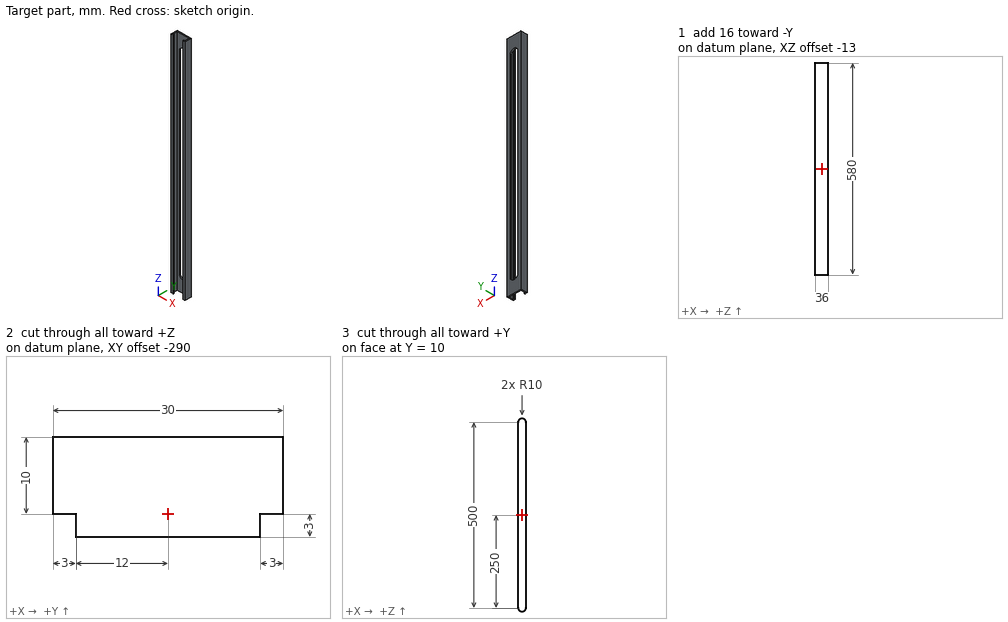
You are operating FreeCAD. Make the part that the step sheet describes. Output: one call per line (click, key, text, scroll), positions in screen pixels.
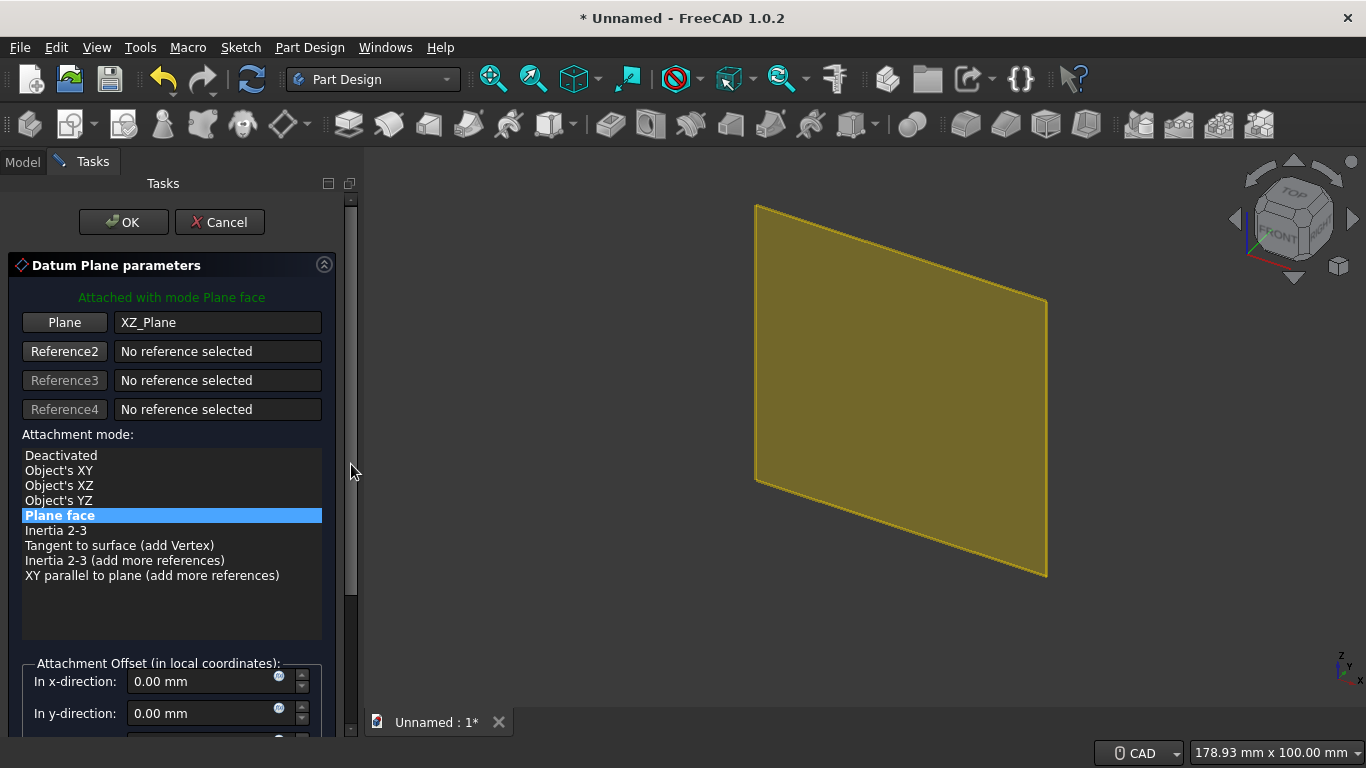
click(124, 222)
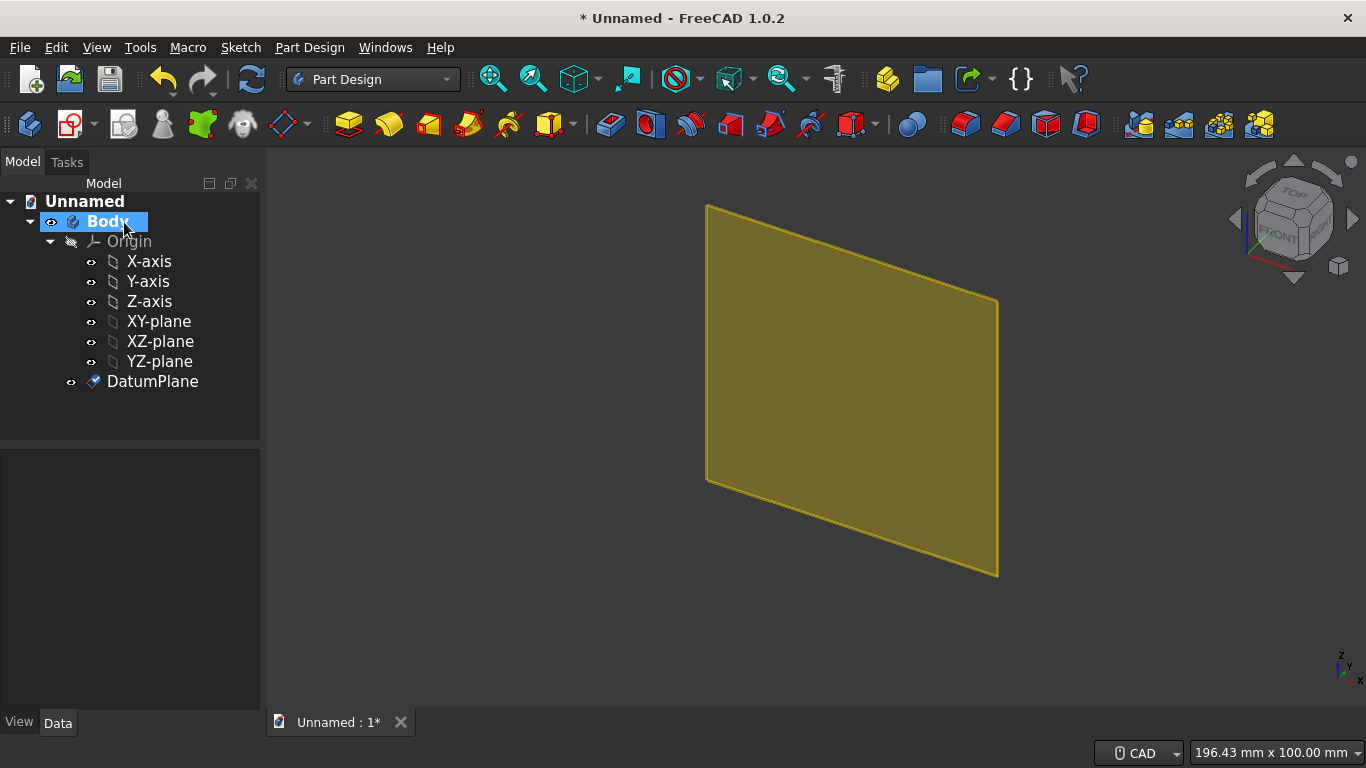
click(116, 382)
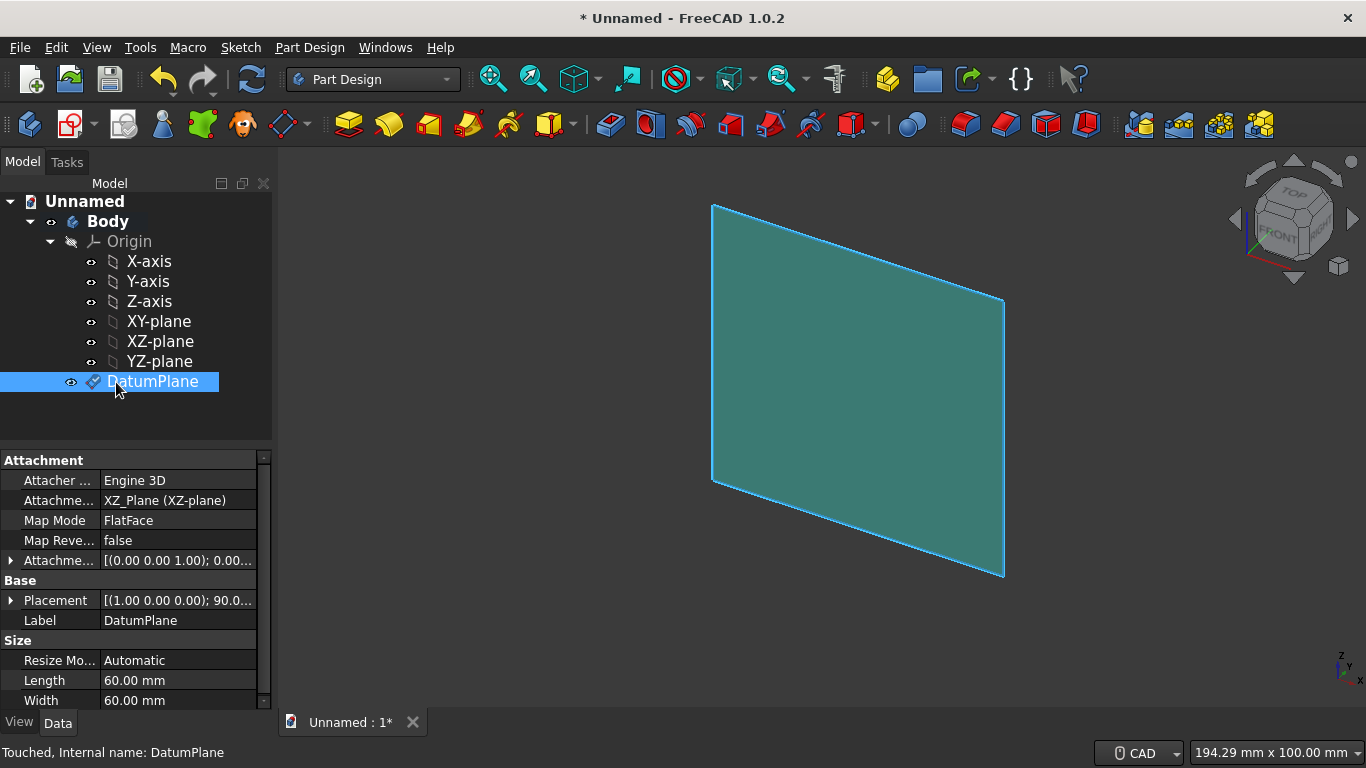
click(70, 124)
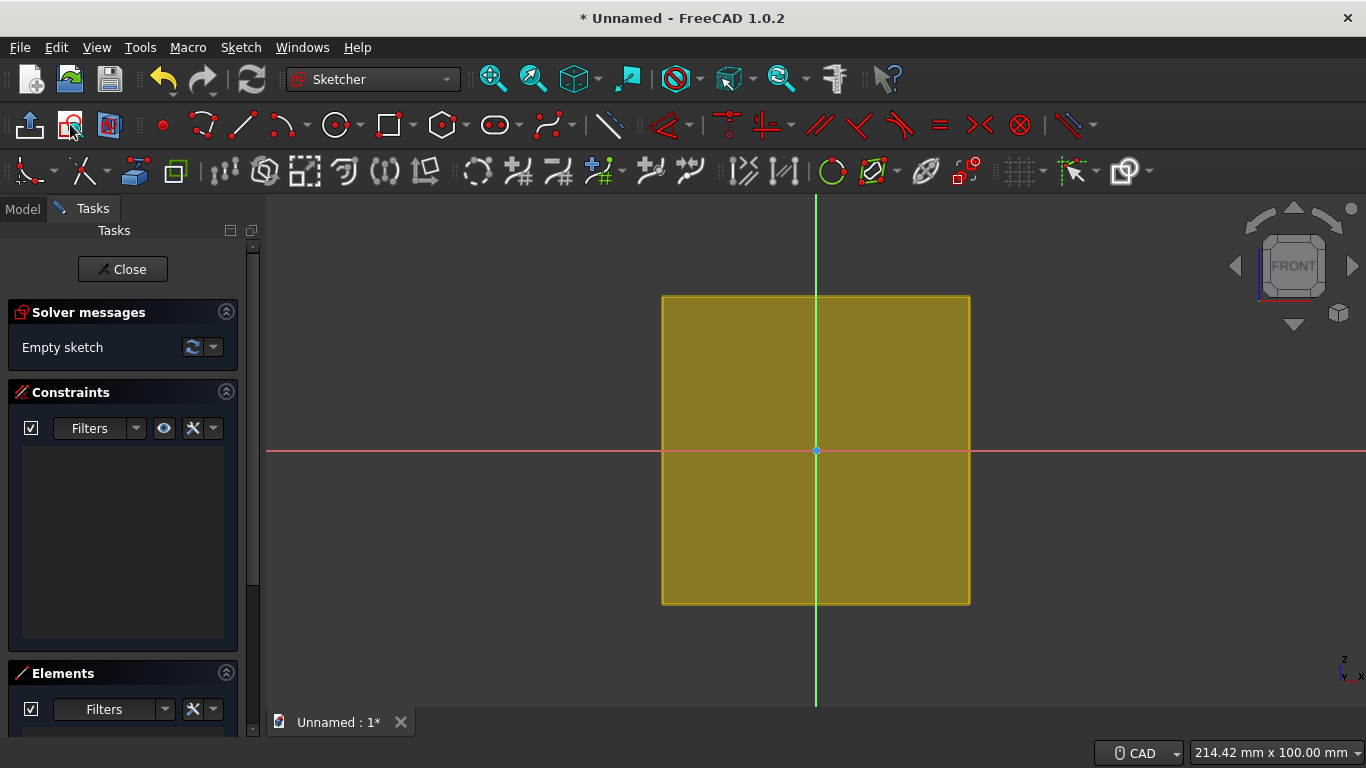
scroll(739, 450, down, 11)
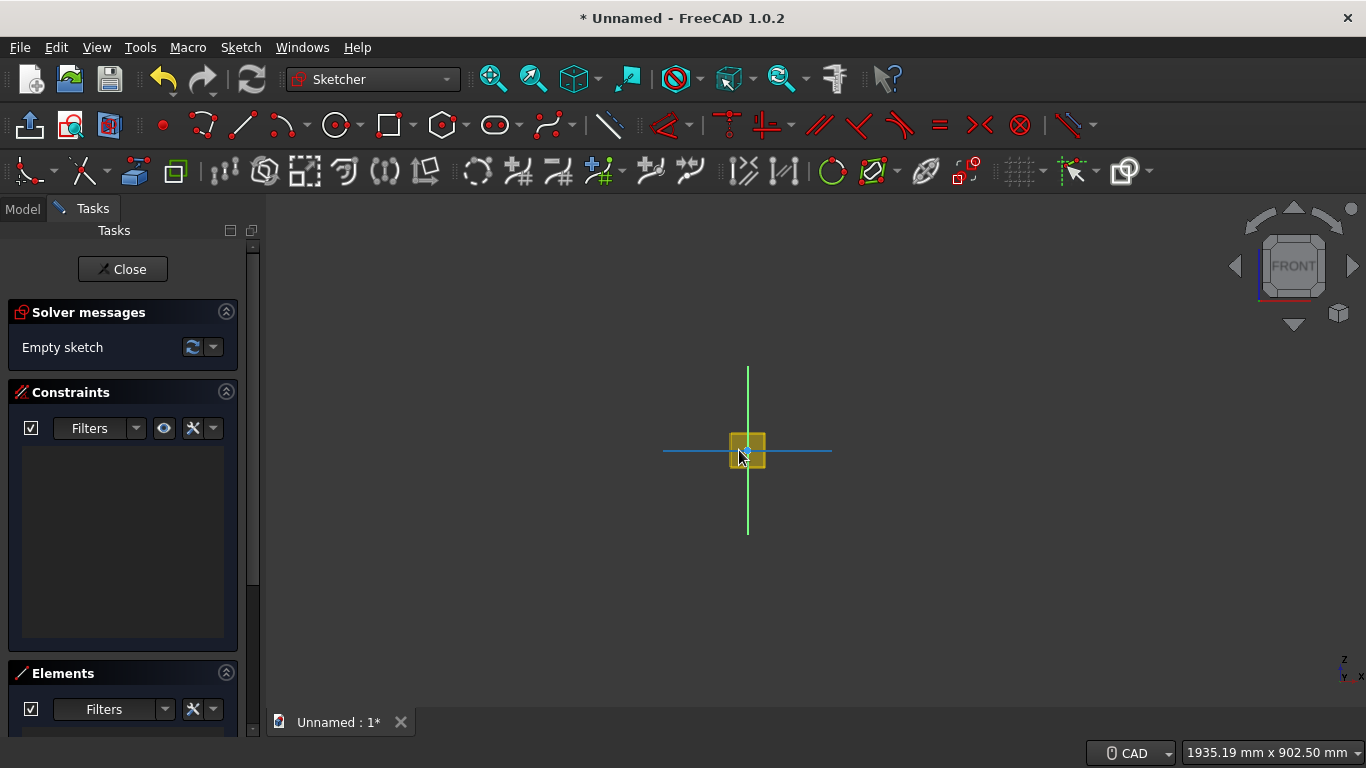
click(416, 126)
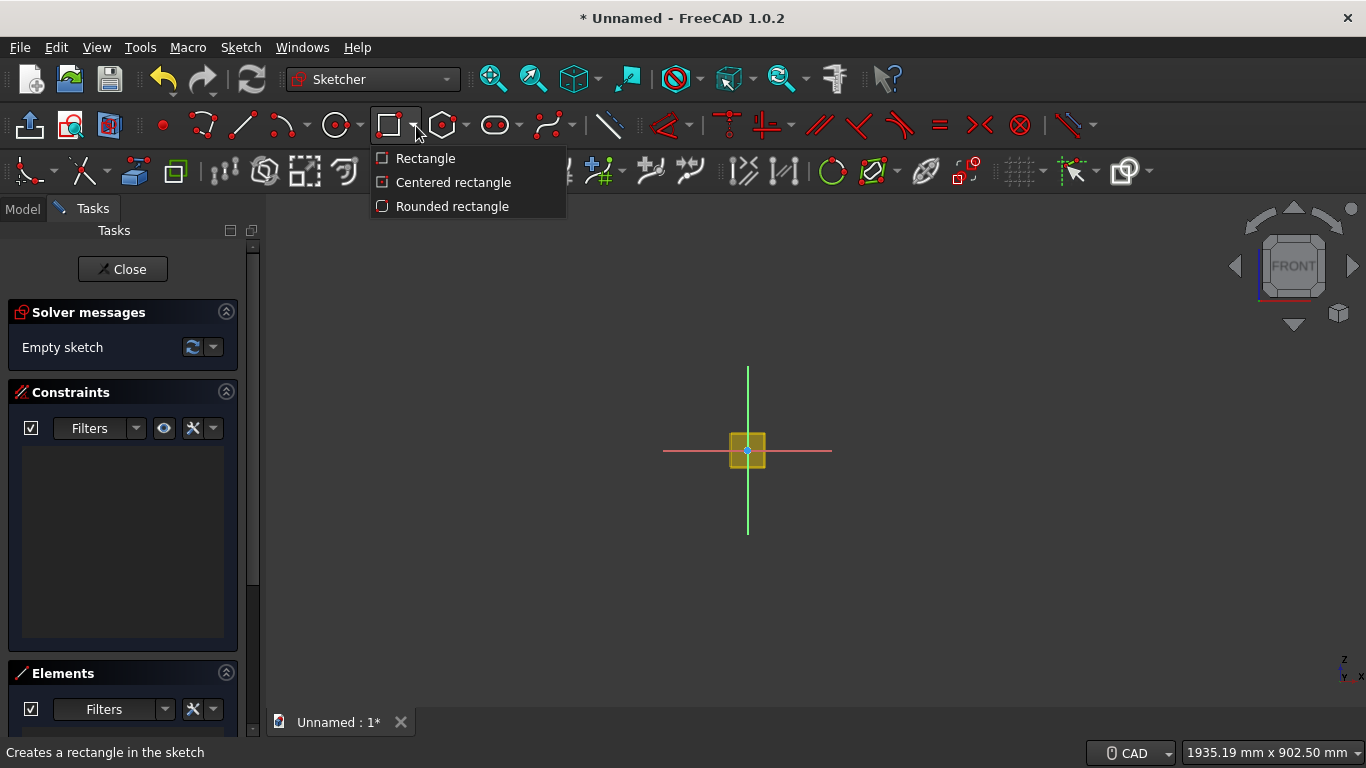
click(468, 182)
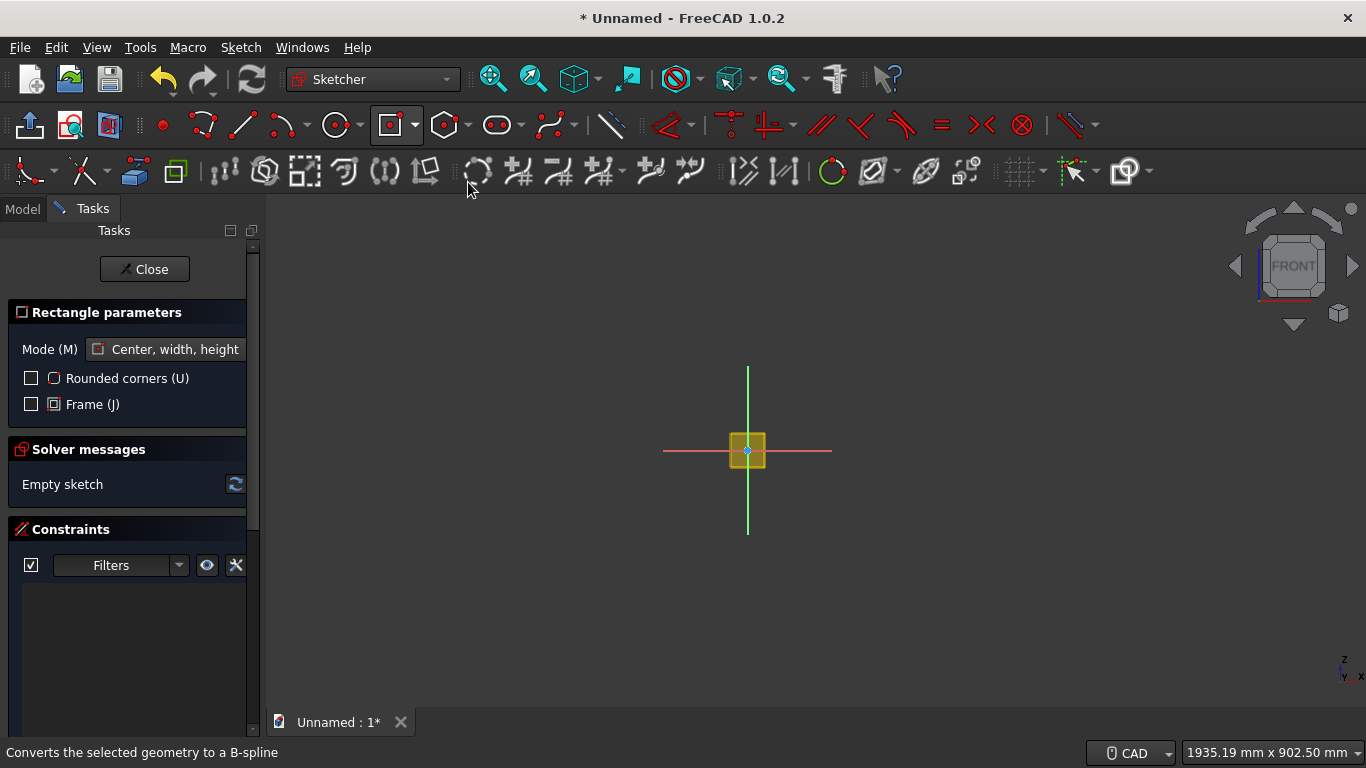
scroll(748, 450, up, 3)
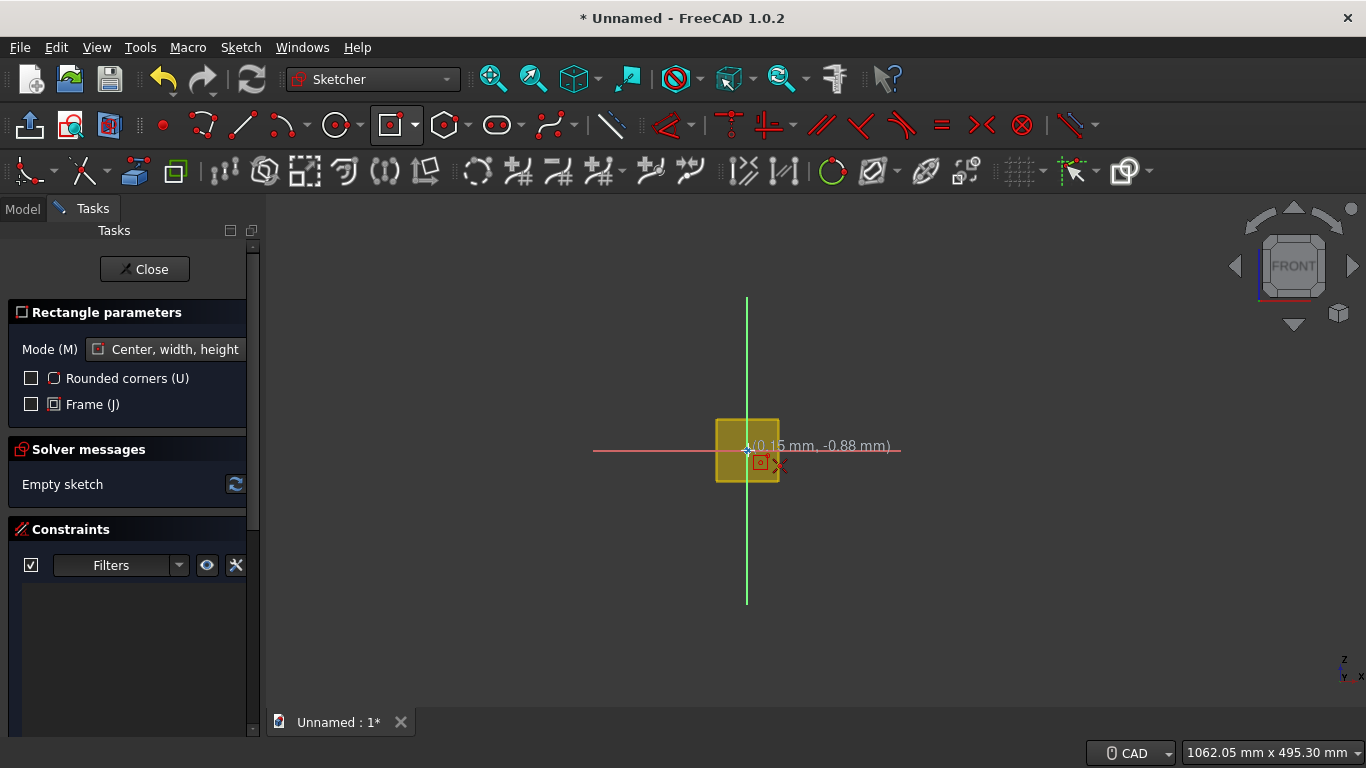
click(747, 450)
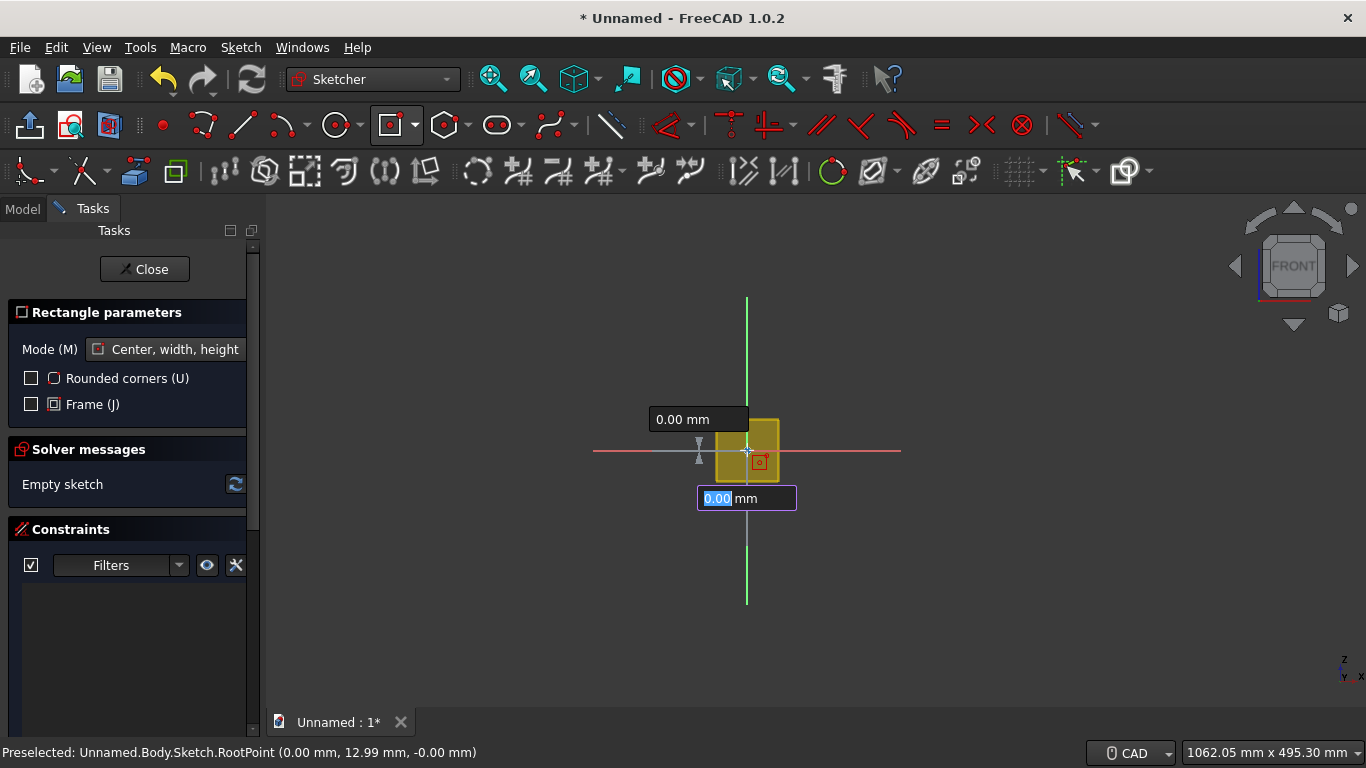
scroll(748, 451, down, 3)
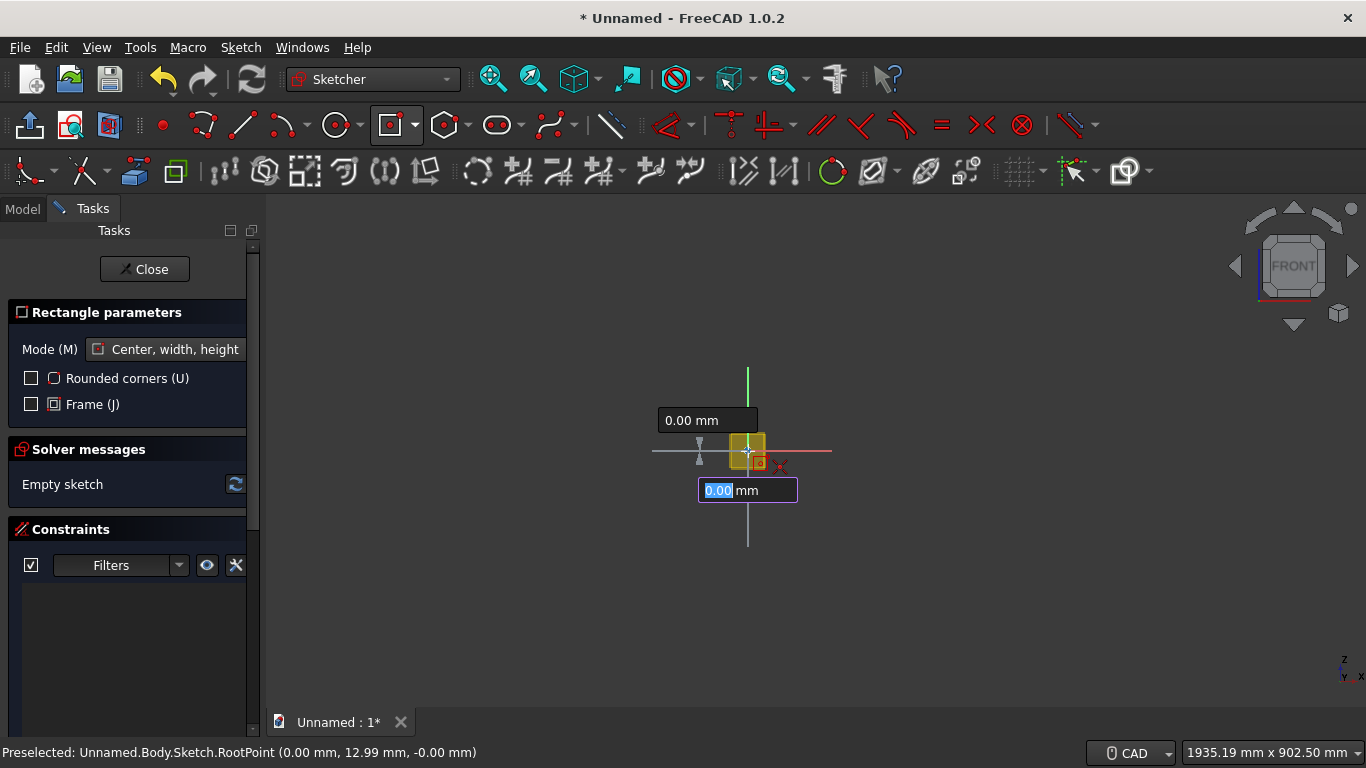
scroll(758, 286, up, 3)